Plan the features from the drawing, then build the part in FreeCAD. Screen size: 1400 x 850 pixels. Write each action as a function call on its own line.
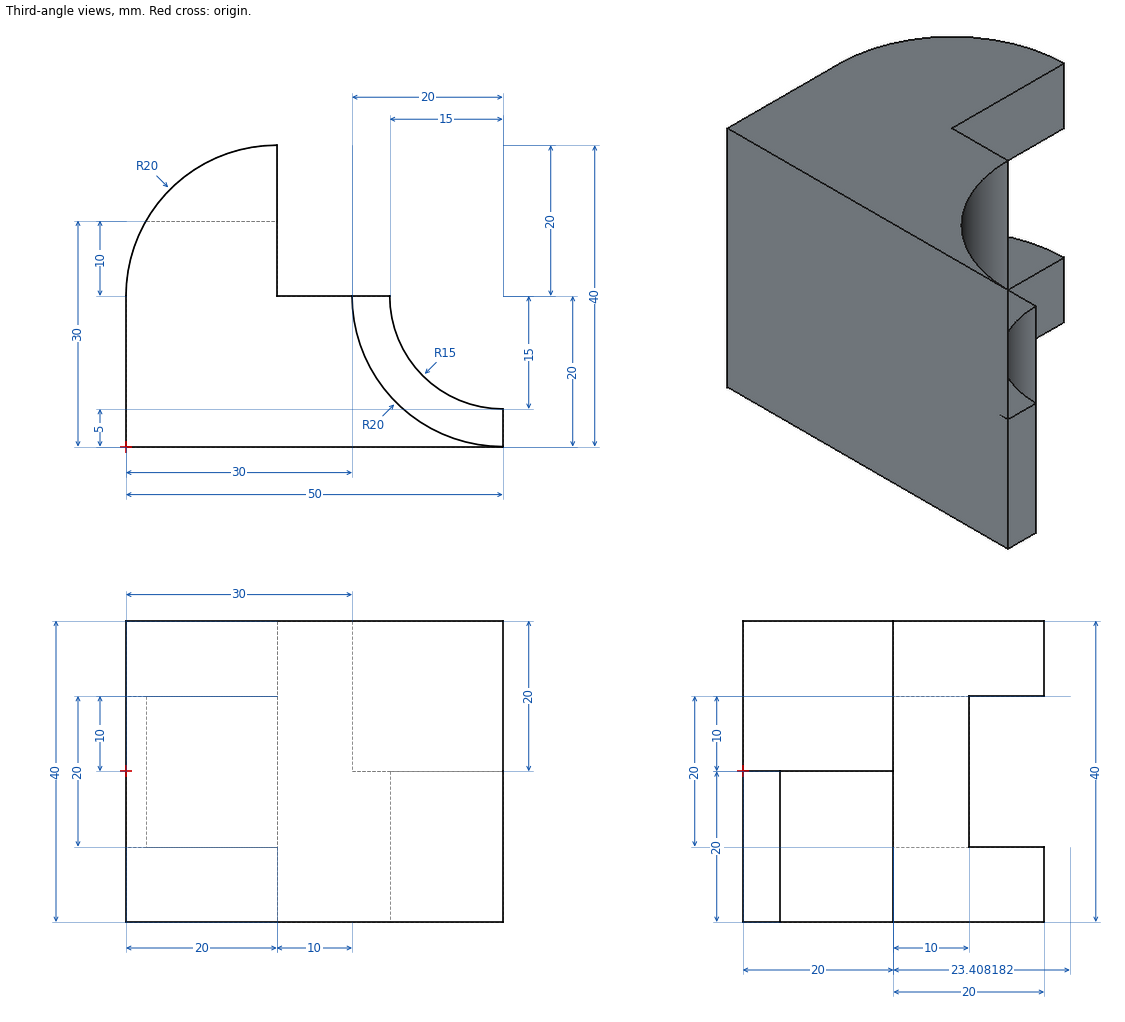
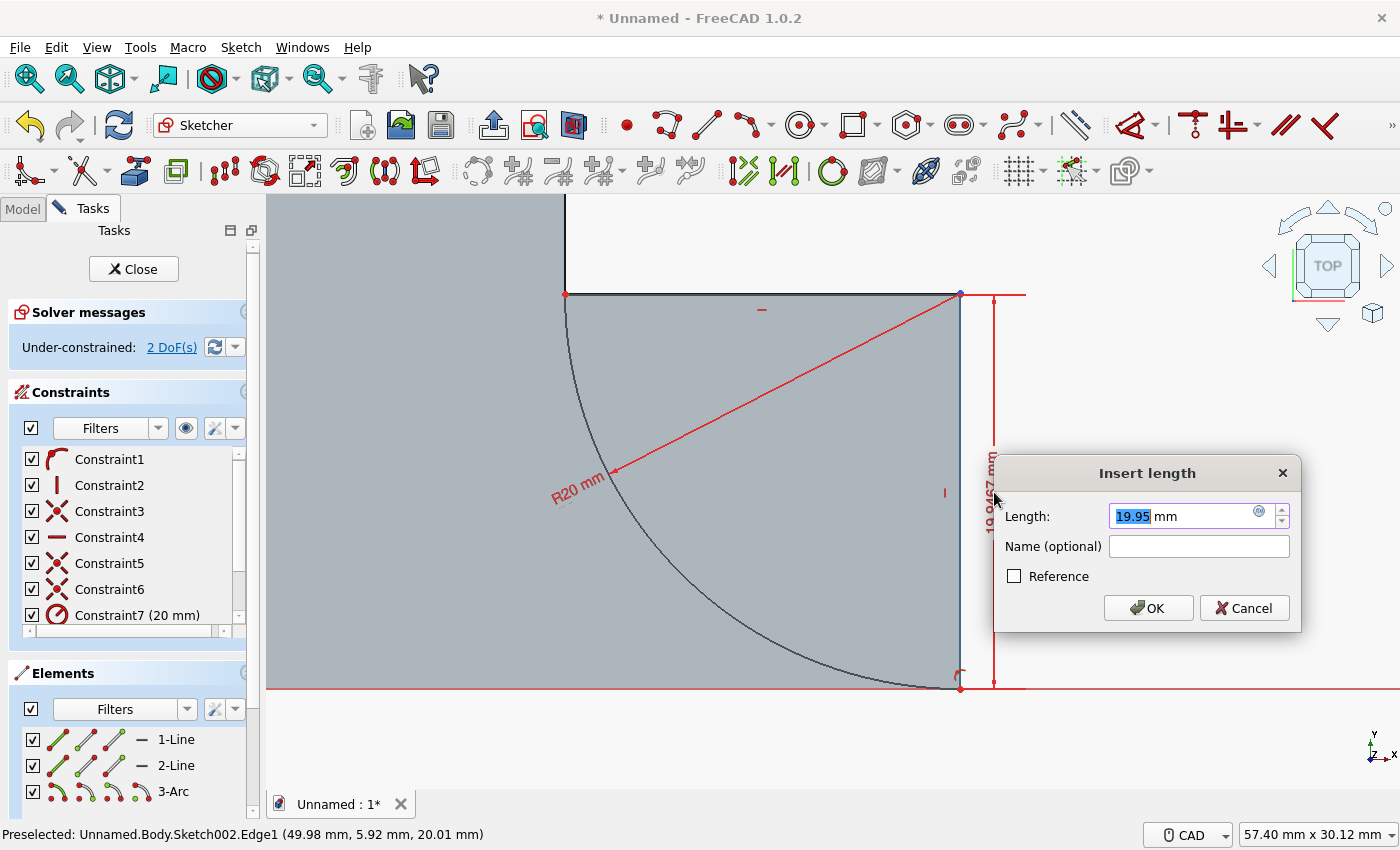
text(20)
key(Return)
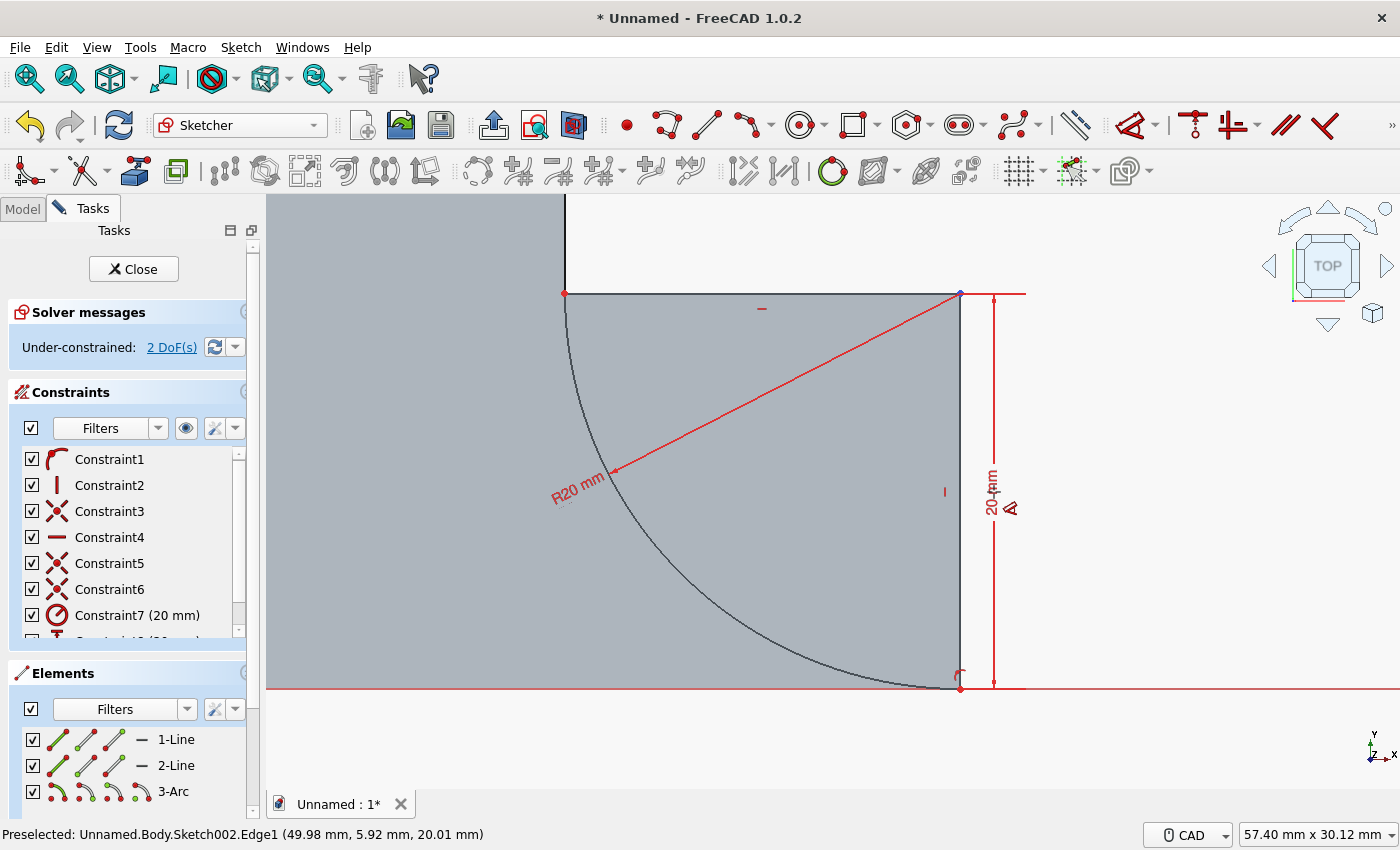
click(841, 294)
click(762, 260)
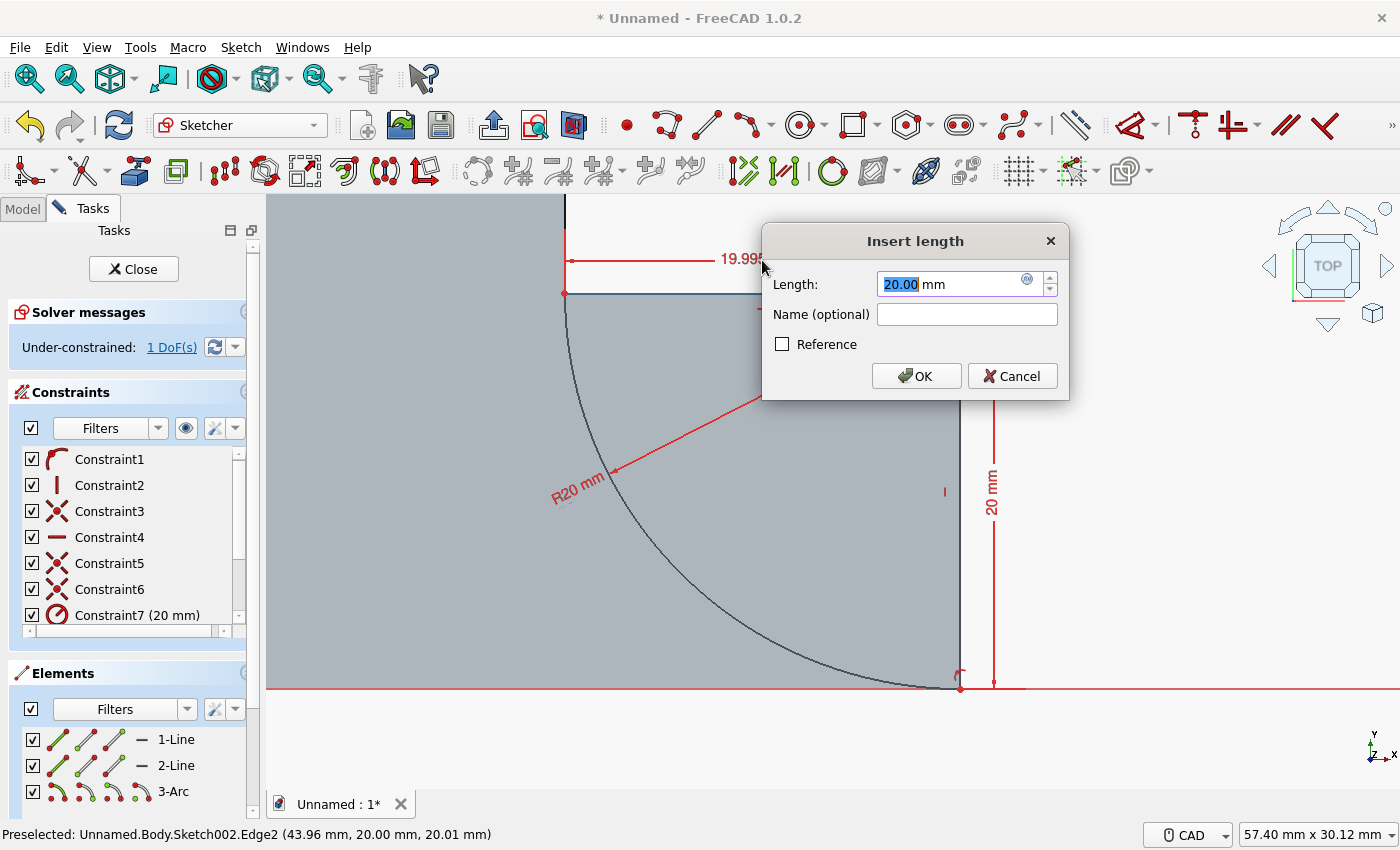
text(20)
key(Return)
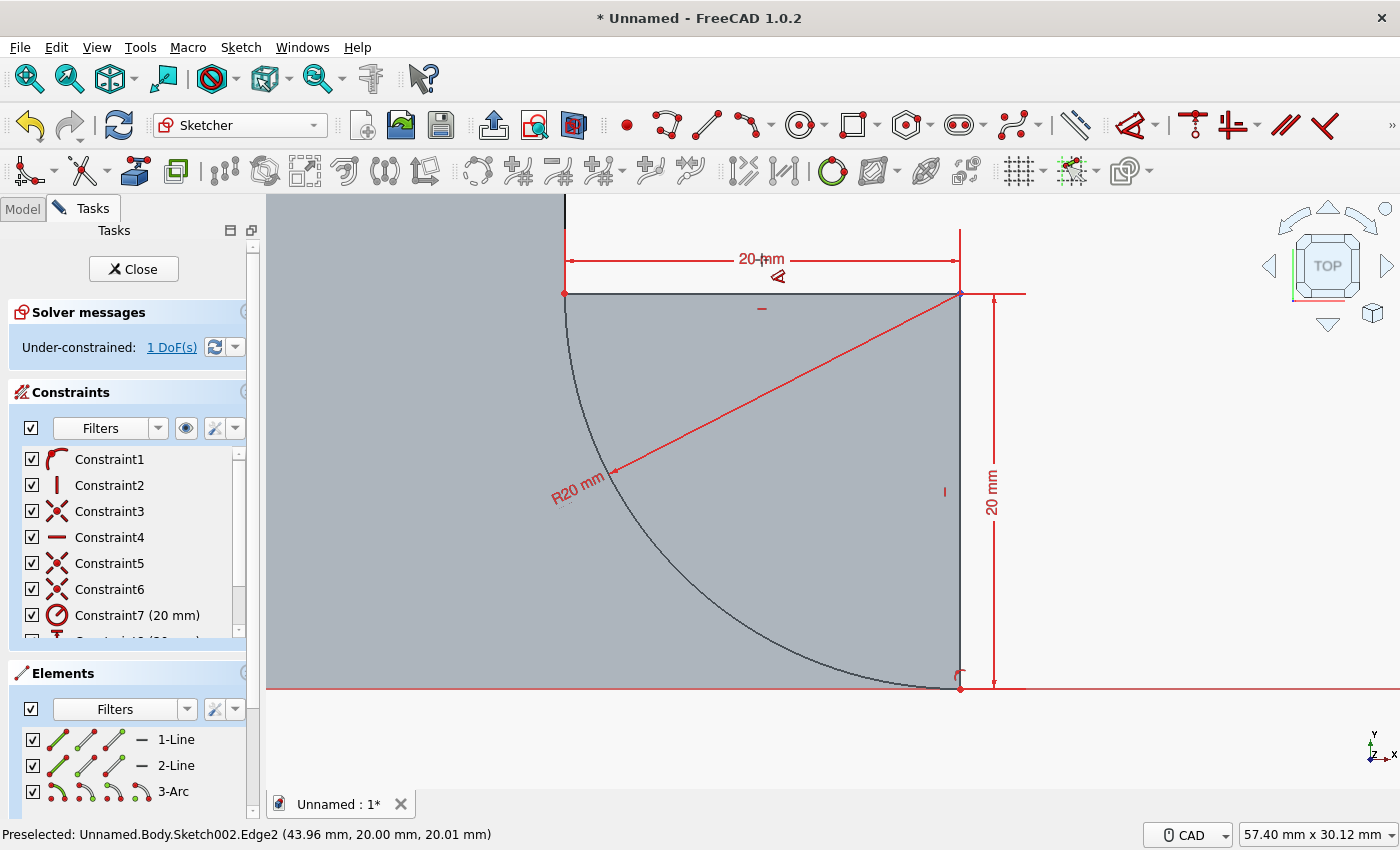
click(960, 689)
click(627, 723)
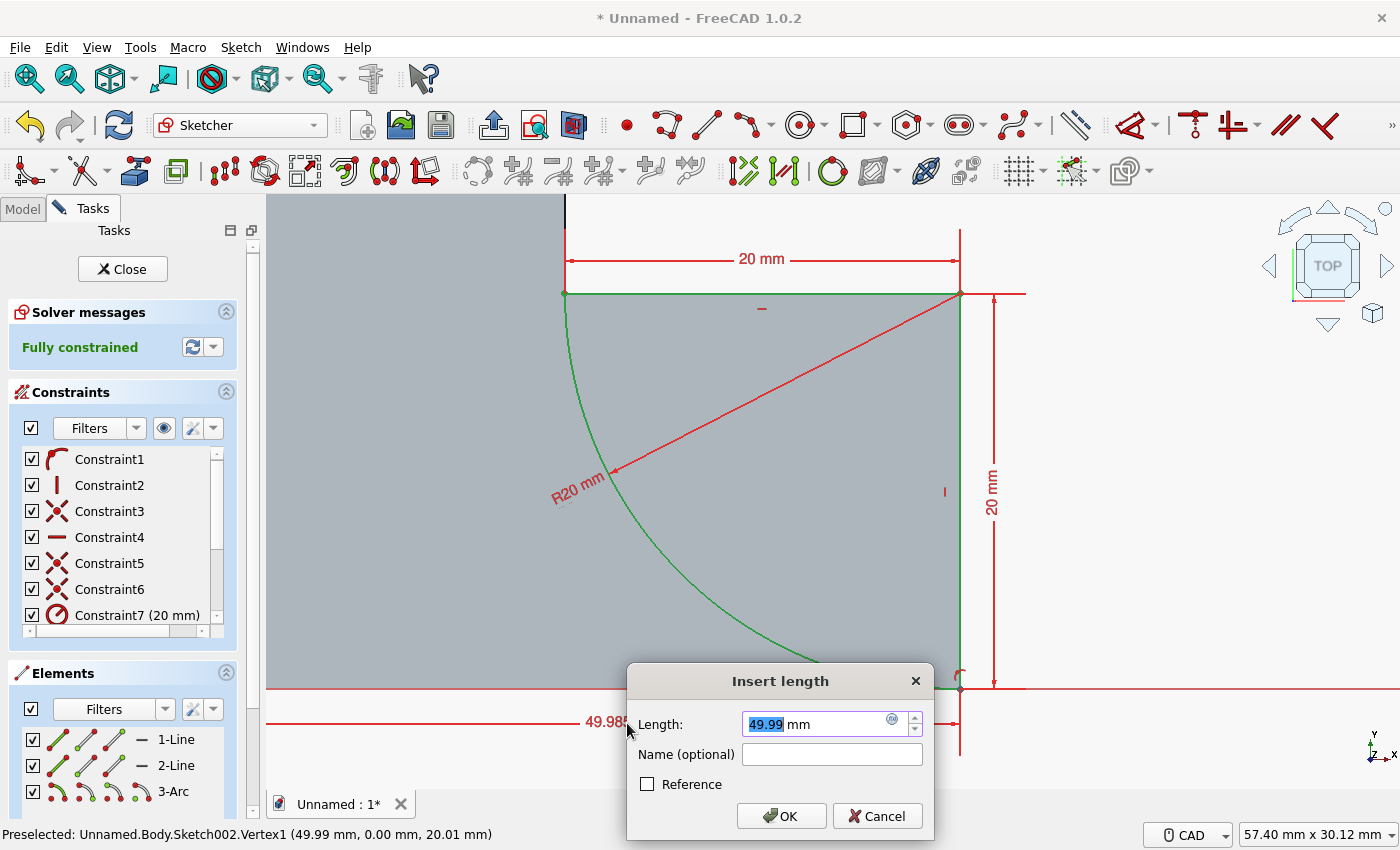
text(50)
key(Return)
key(Escape)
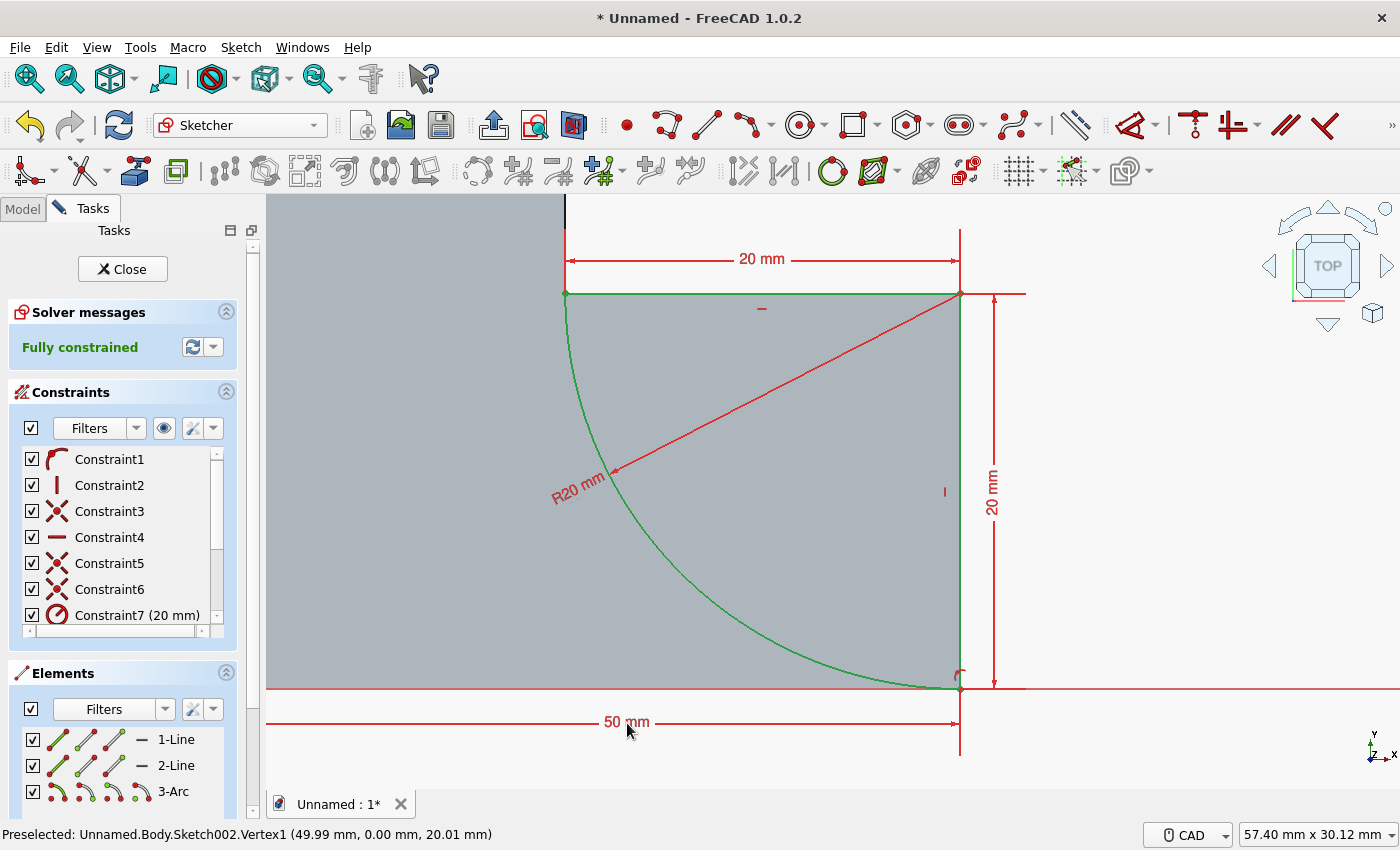
click(123, 269)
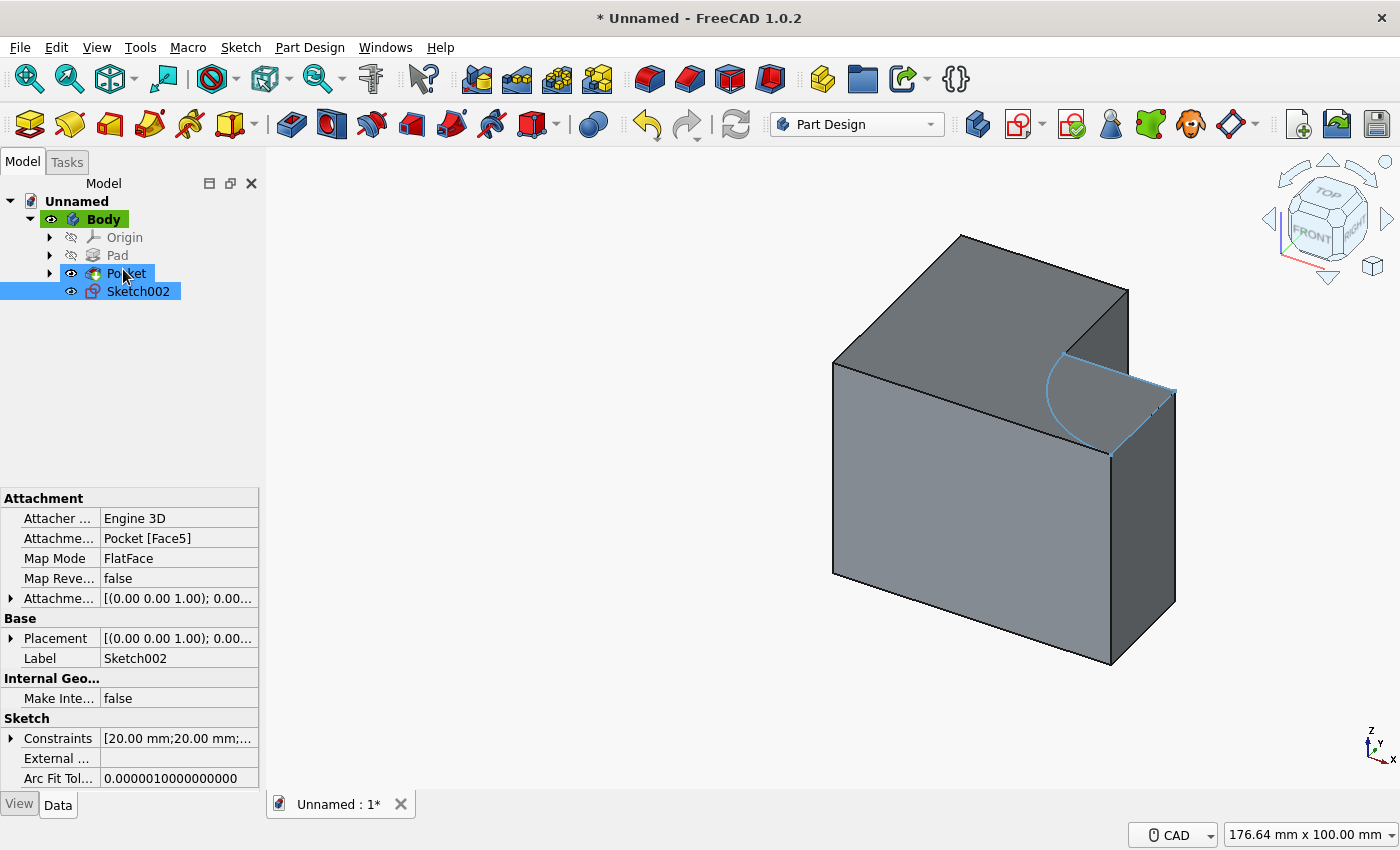
click(292, 124)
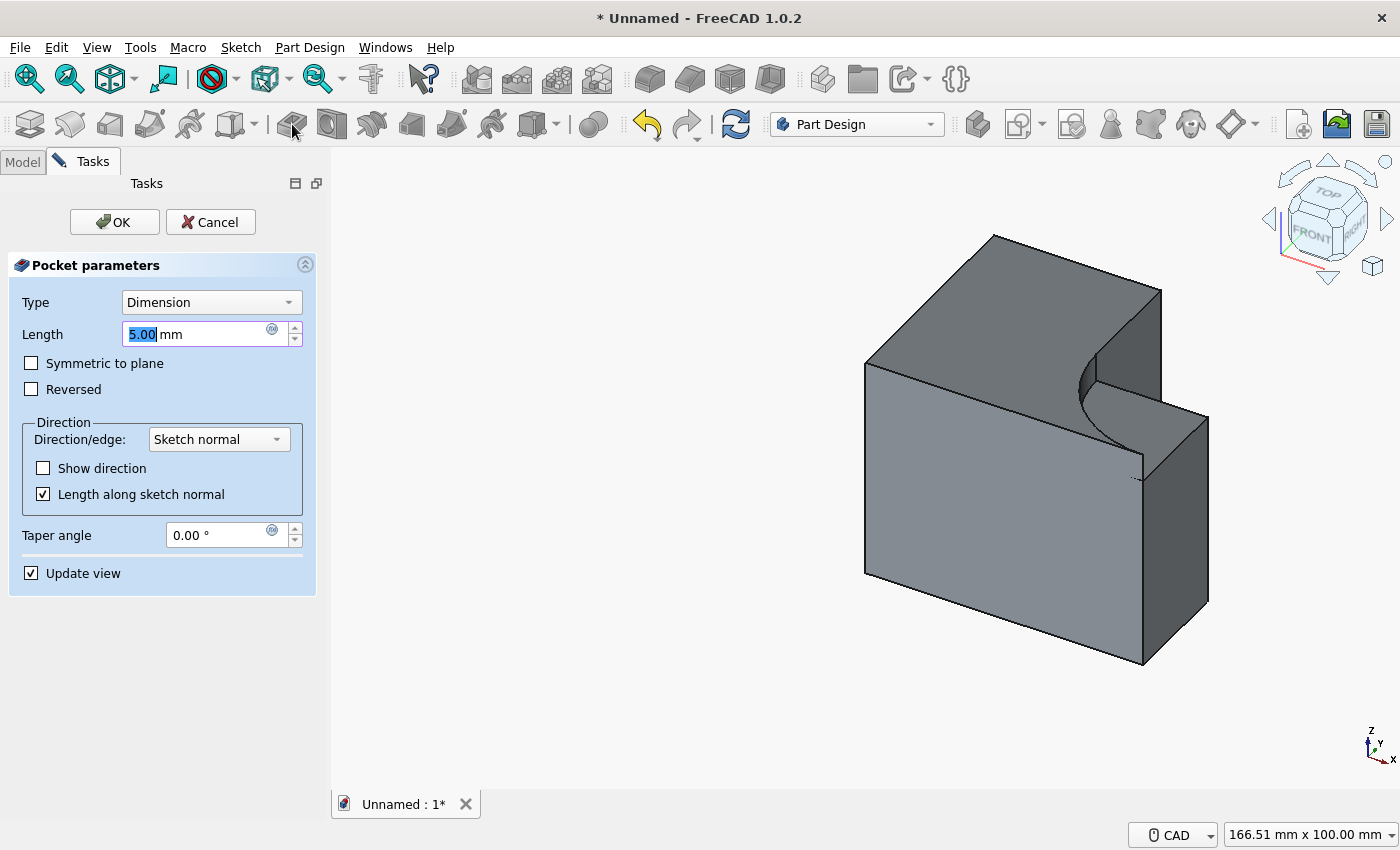
text(20)
key(Tab)